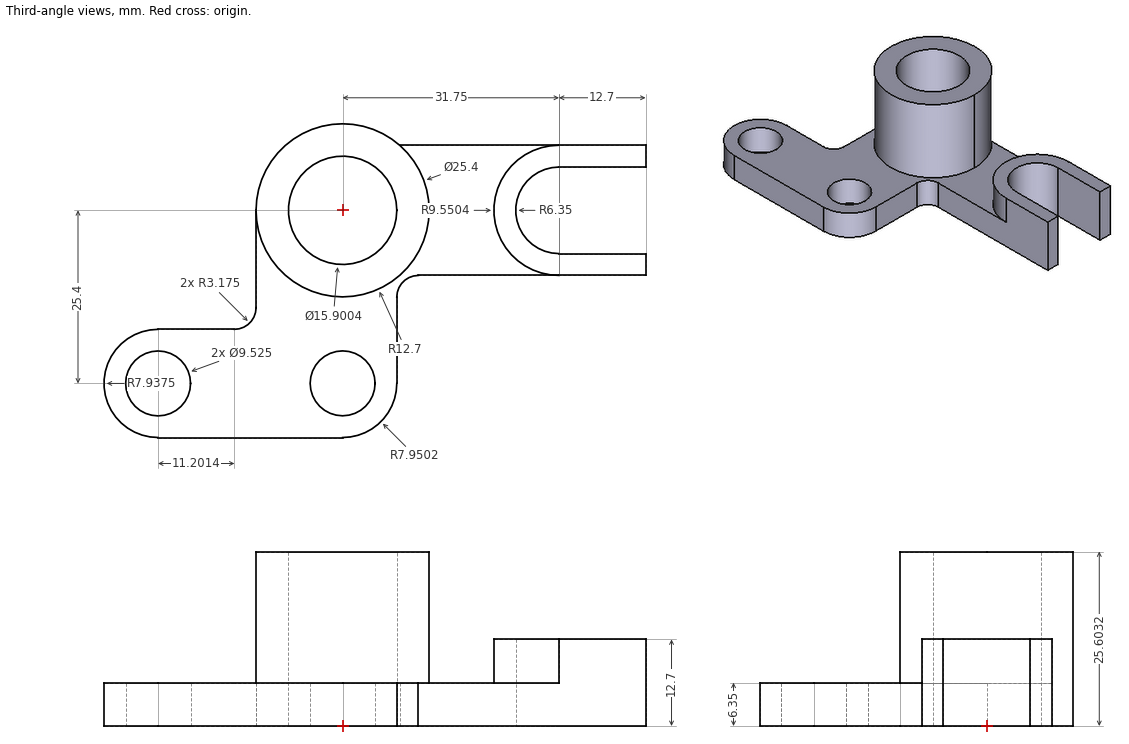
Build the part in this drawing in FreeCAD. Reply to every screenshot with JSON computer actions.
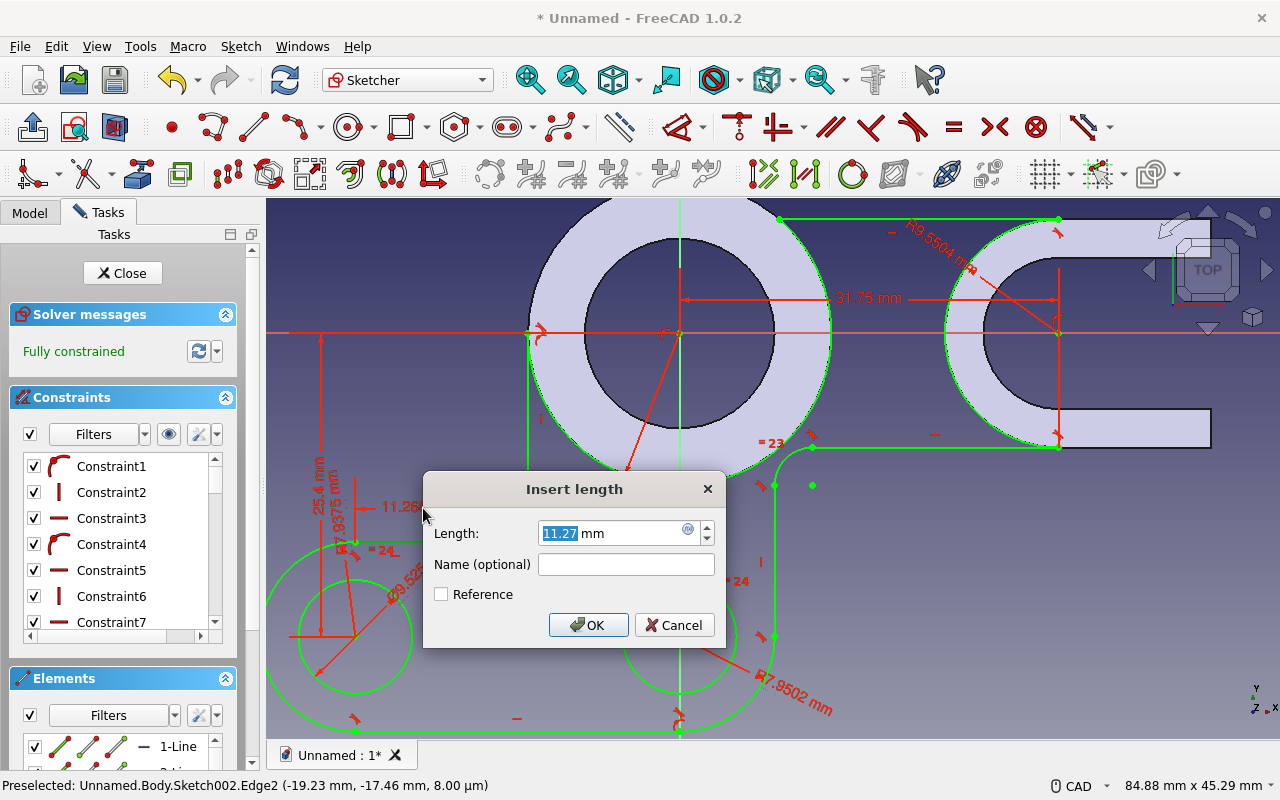
{"action": "type", "text": "11.2014"}
{"action": "key", "text": "Return"}
{"action": "key", "text": "Escape"}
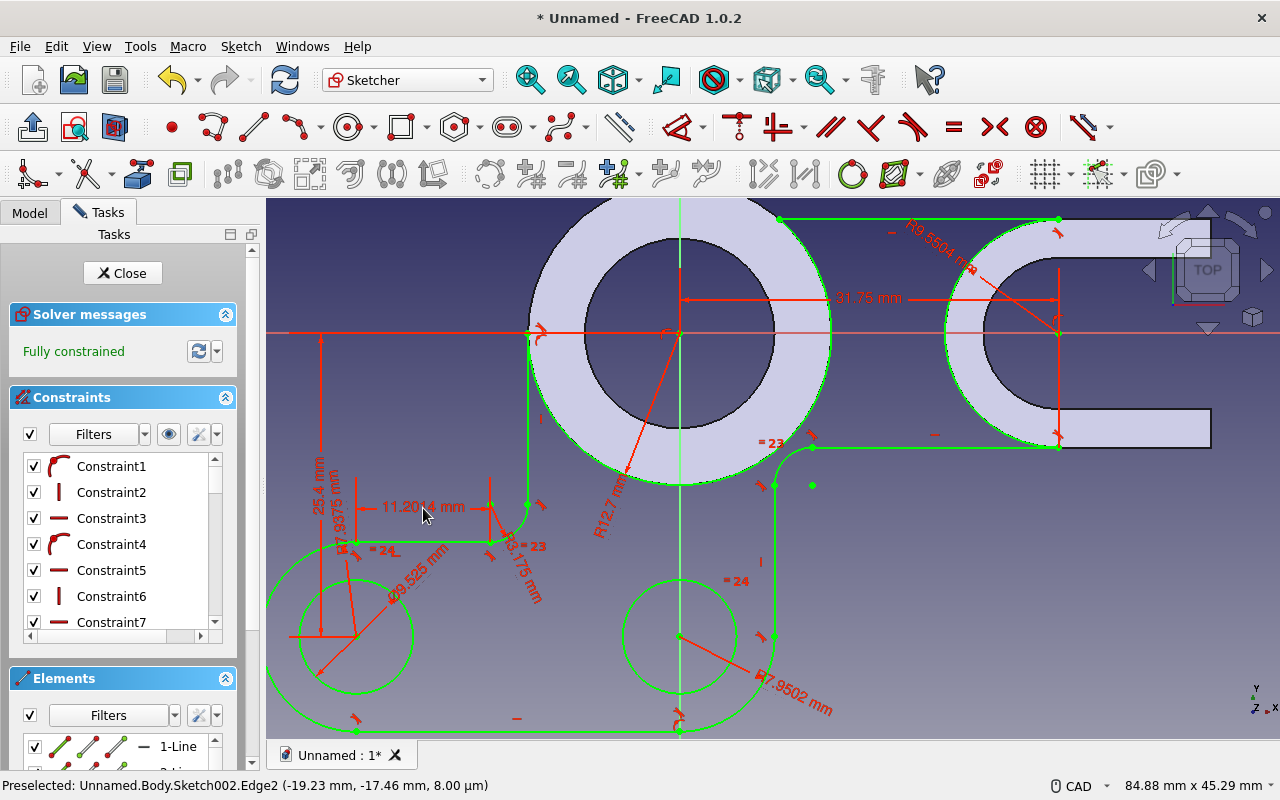
{"action": "left_click", "coordinate": [123, 273]}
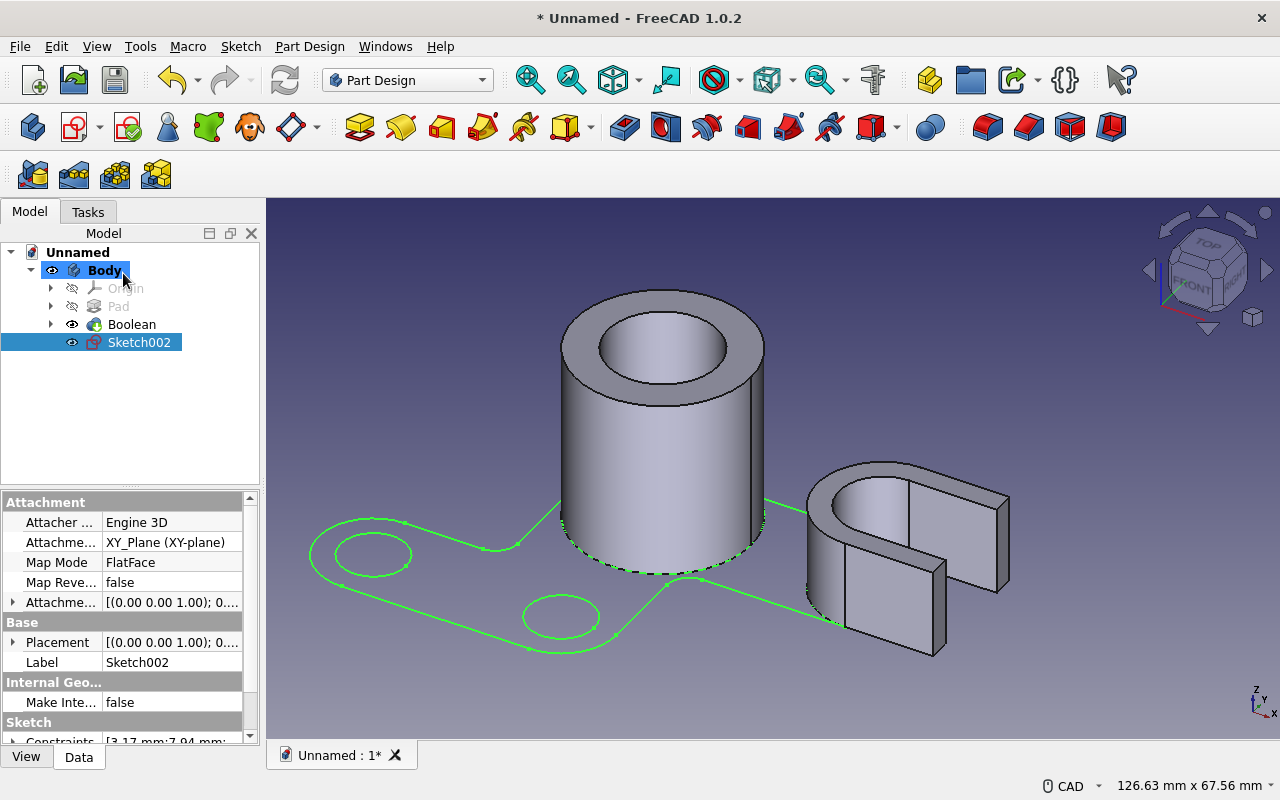
{"action": "left_click", "coordinate": [360, 128]}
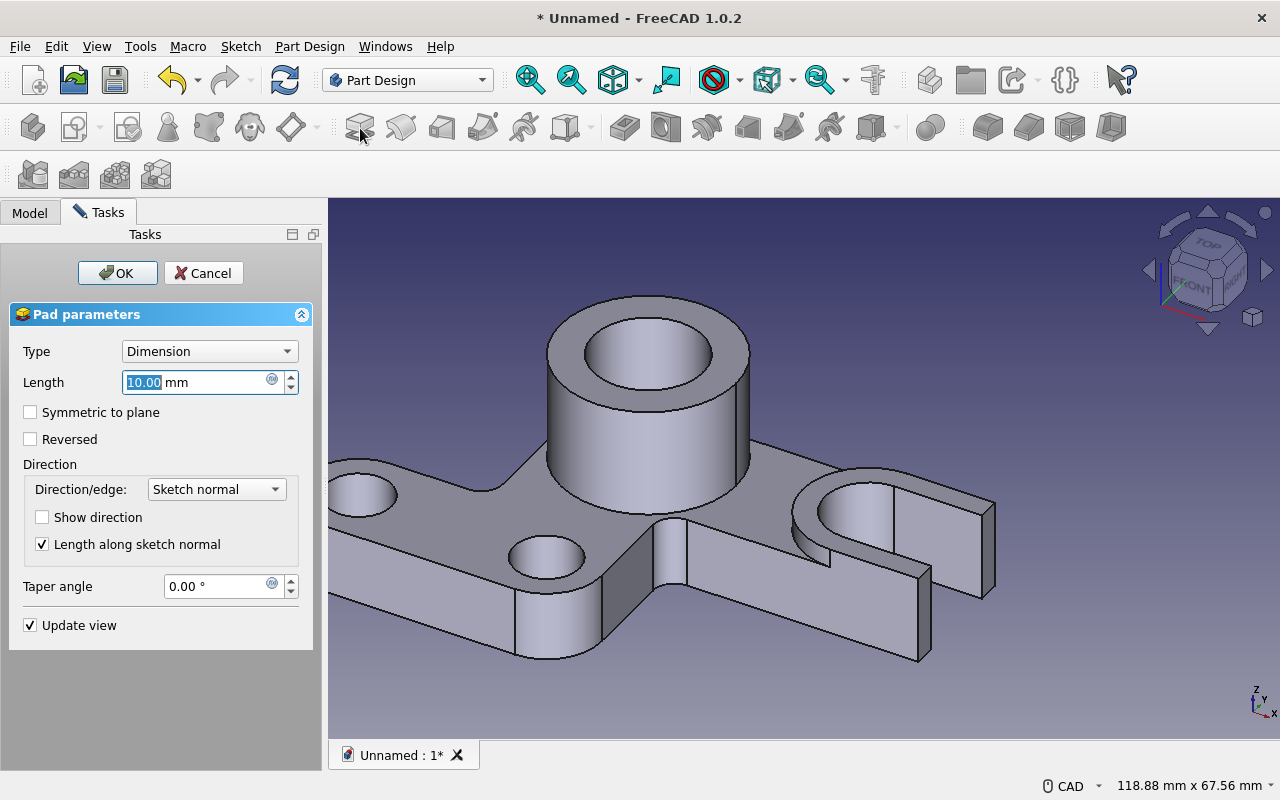
{"action": "type", "text": "6.35"}
{"action": "key", "text": "Tab"}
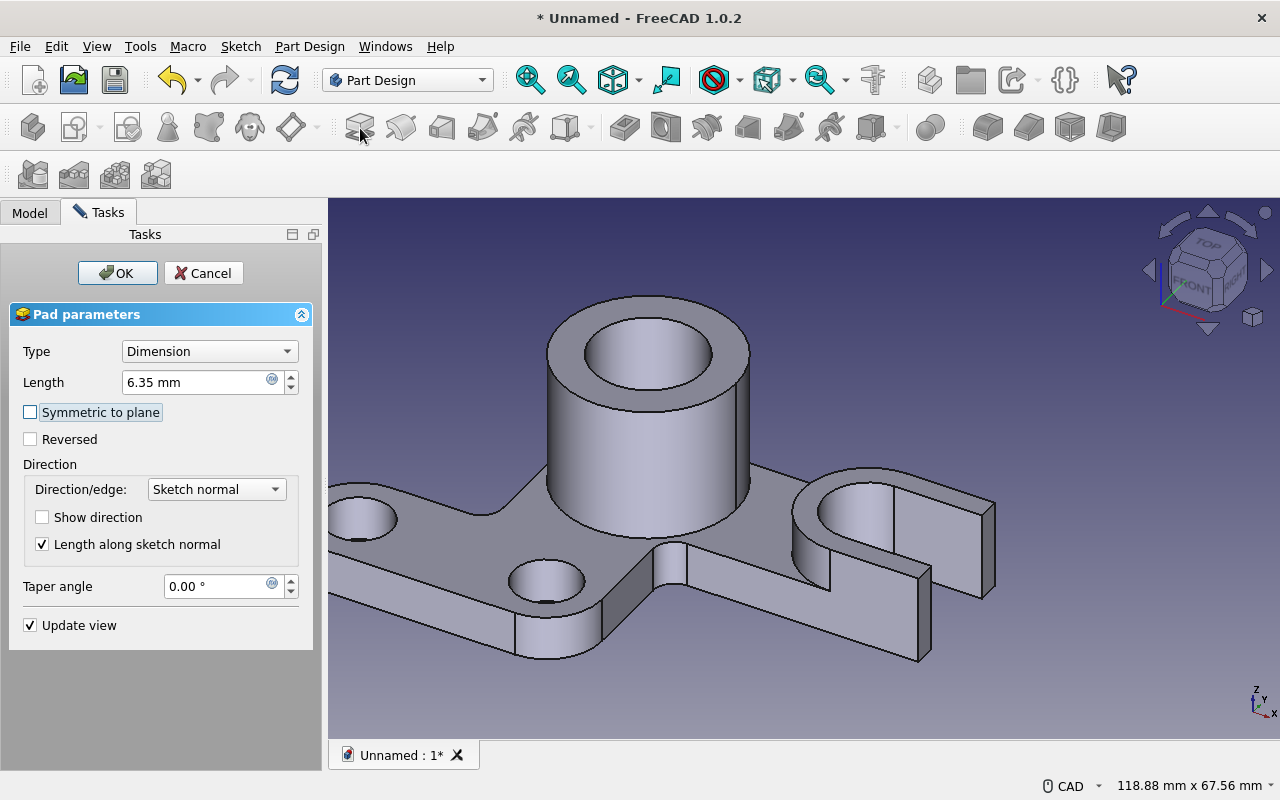
{"action": "left_click", "coordinate": [118, 273]}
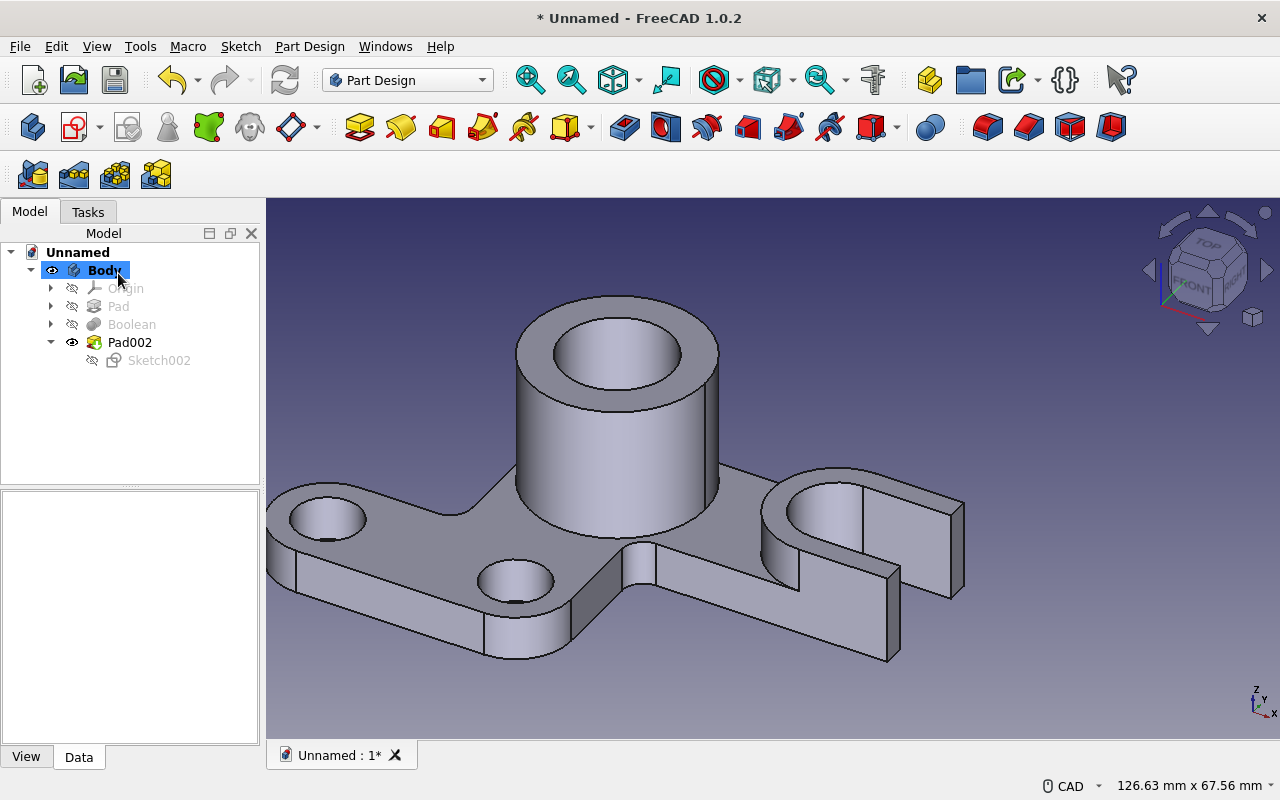
{"action": "key", "text": "0"}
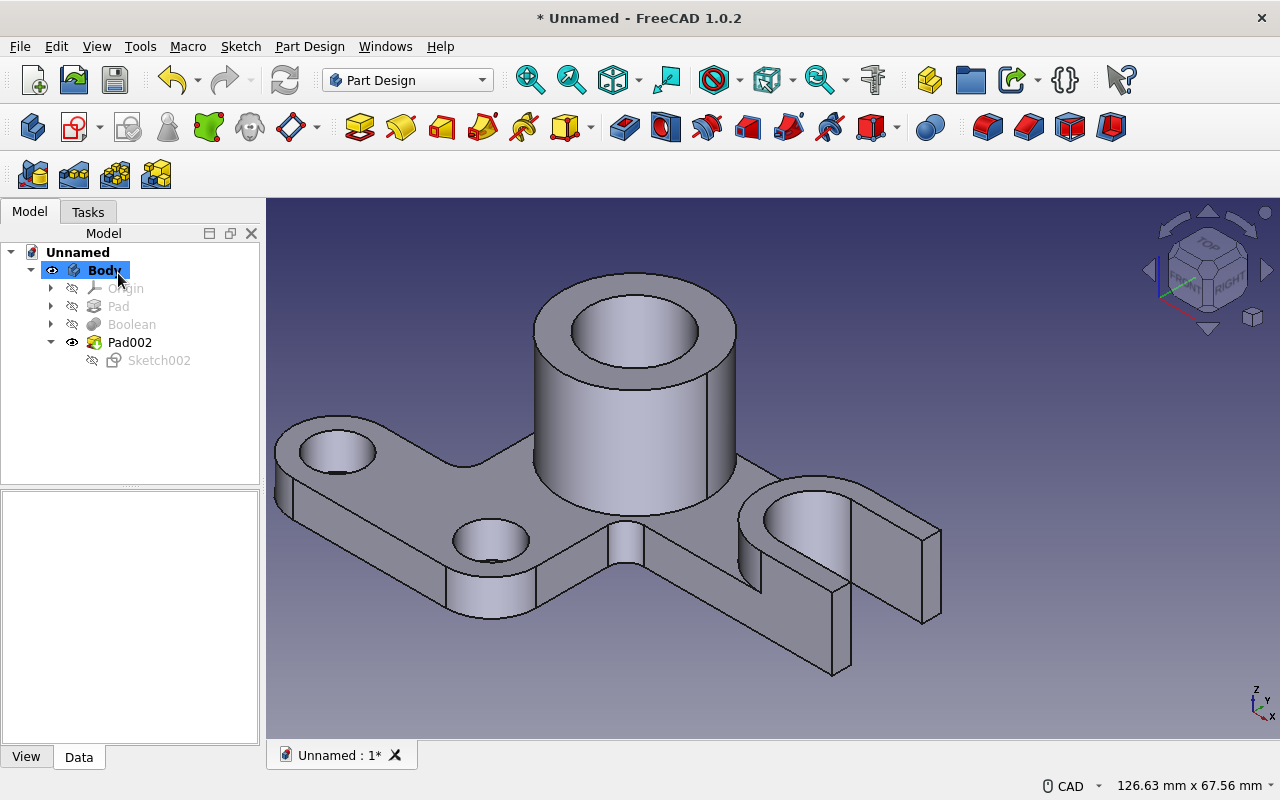
{"action": "left_click", "coordinate": [531, 80]}